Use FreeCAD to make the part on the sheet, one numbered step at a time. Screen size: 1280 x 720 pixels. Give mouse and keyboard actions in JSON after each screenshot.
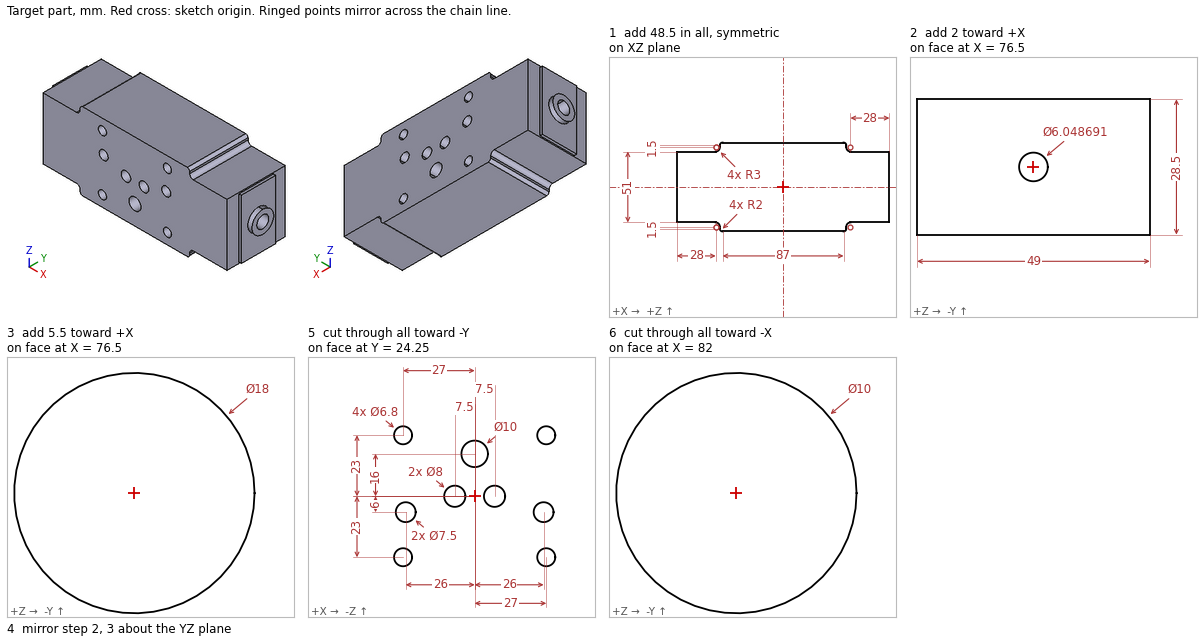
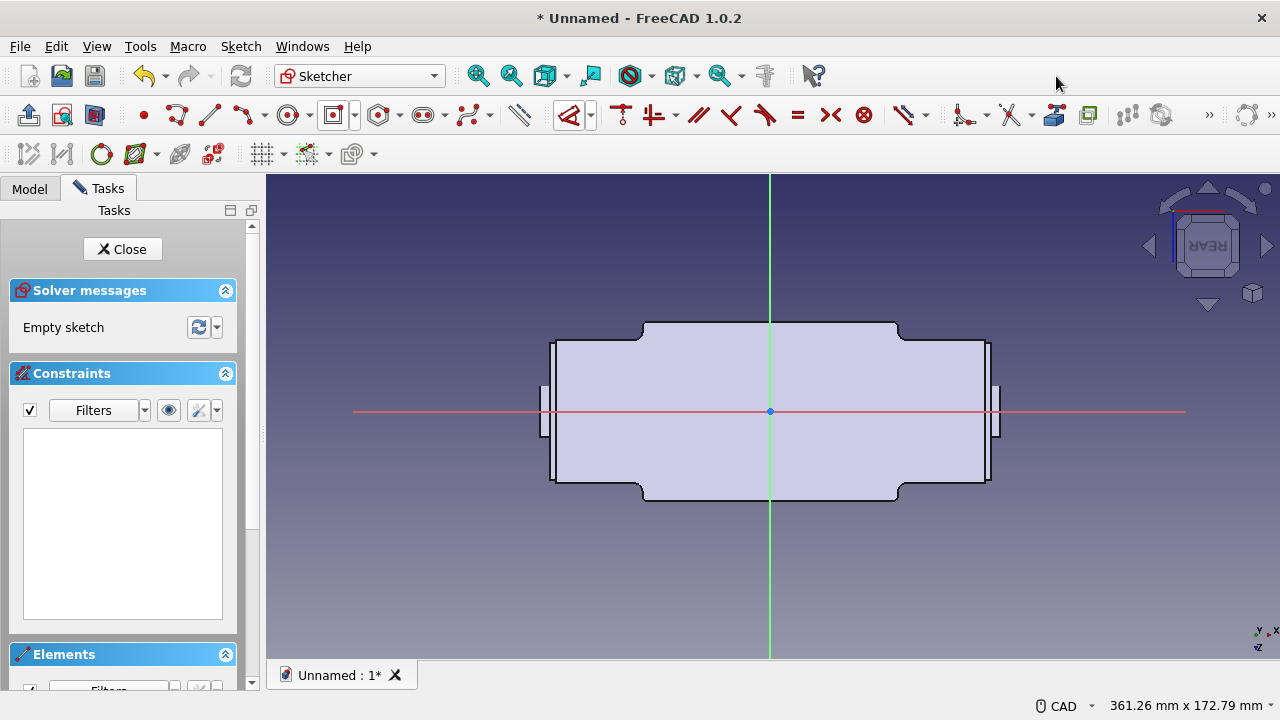
{"action": "scroll", "coordinate": [824, 408], "scroll_direction": "up", "scroll_amount": 4}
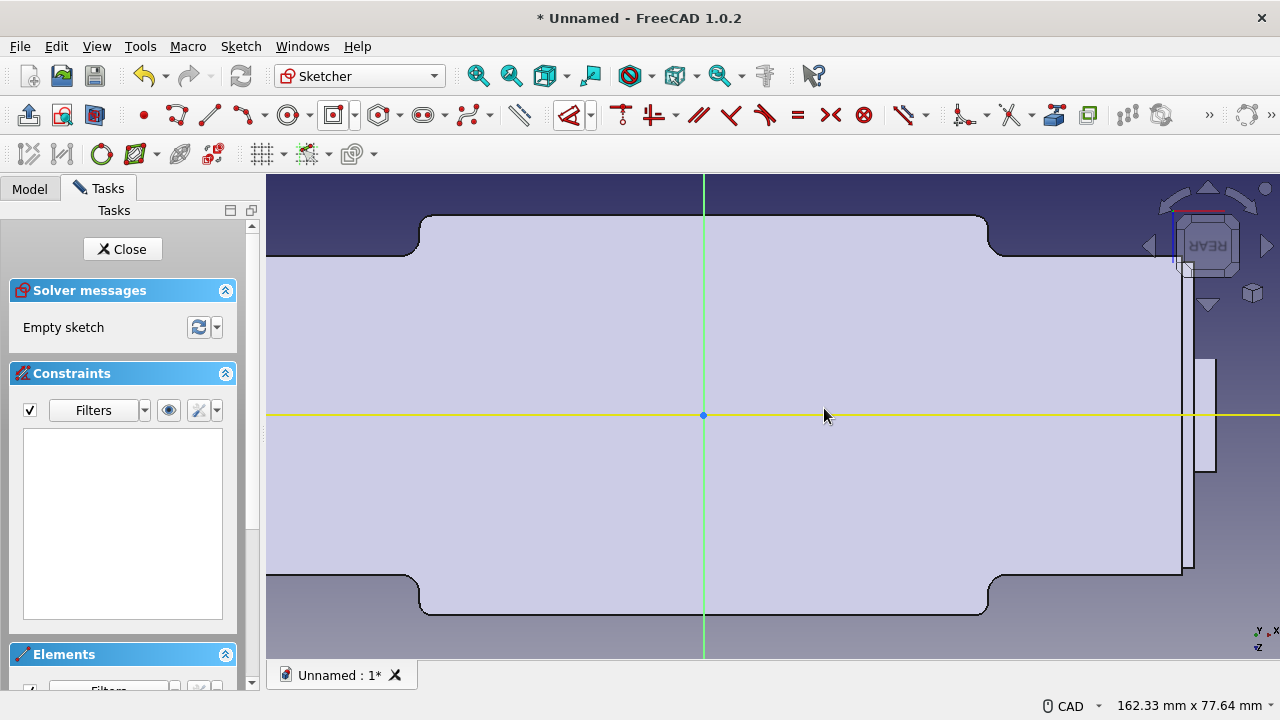
{"action": "key", "text": "g c"}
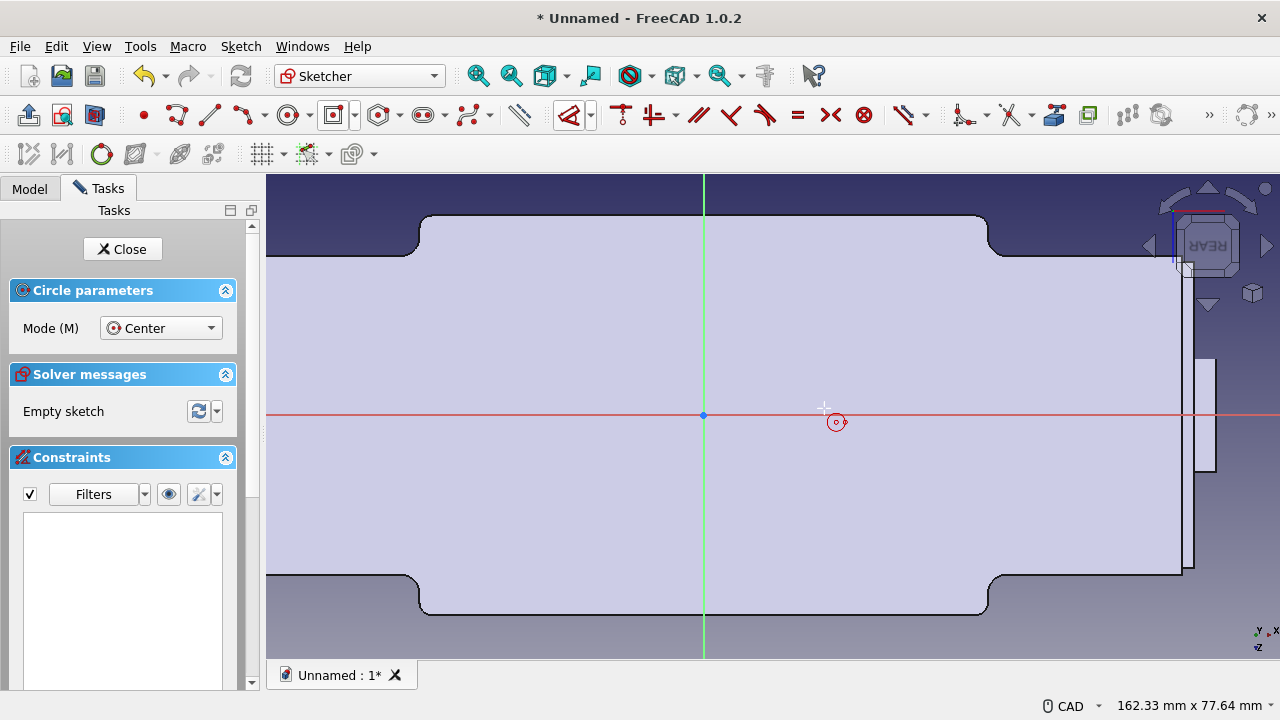
{"action": "left_click", "coordinate": [535, 272]}
{"action": "left_click", "coordinate": [550, 257]}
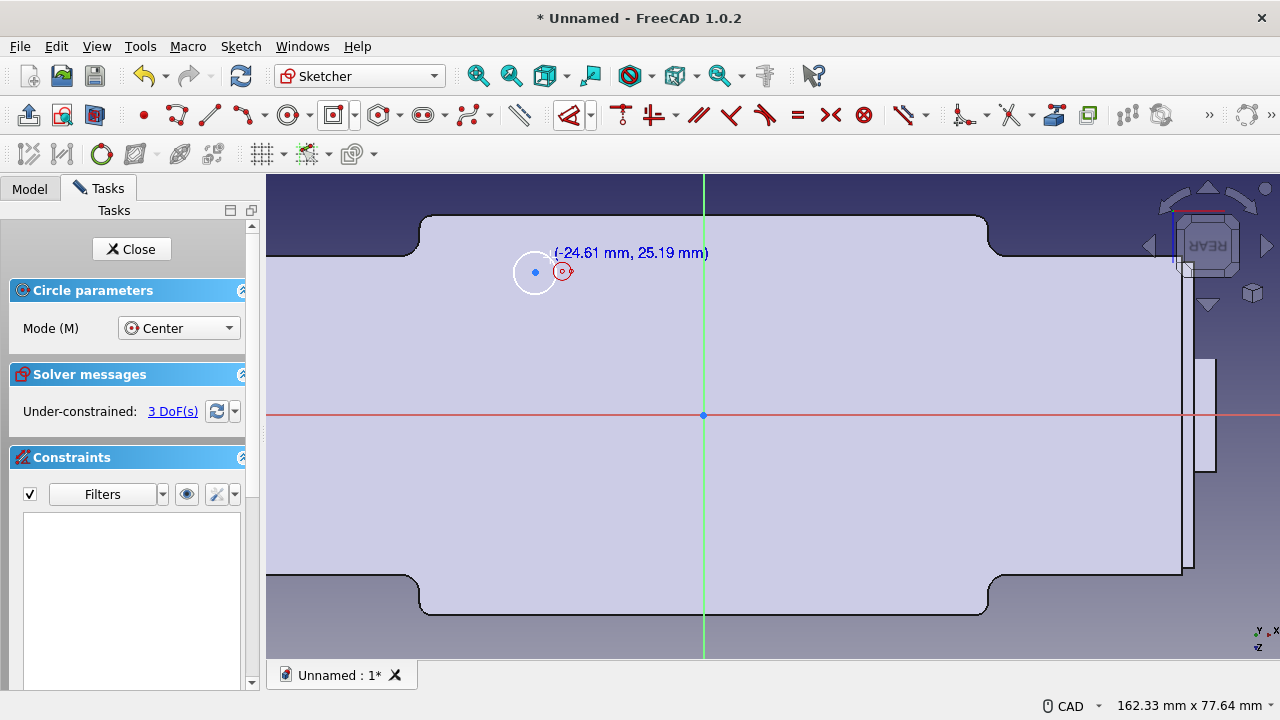
{"action": "left_click", "coordinate": [704, 315]}
{"action": "left_click", "coordinate": [726, 293]}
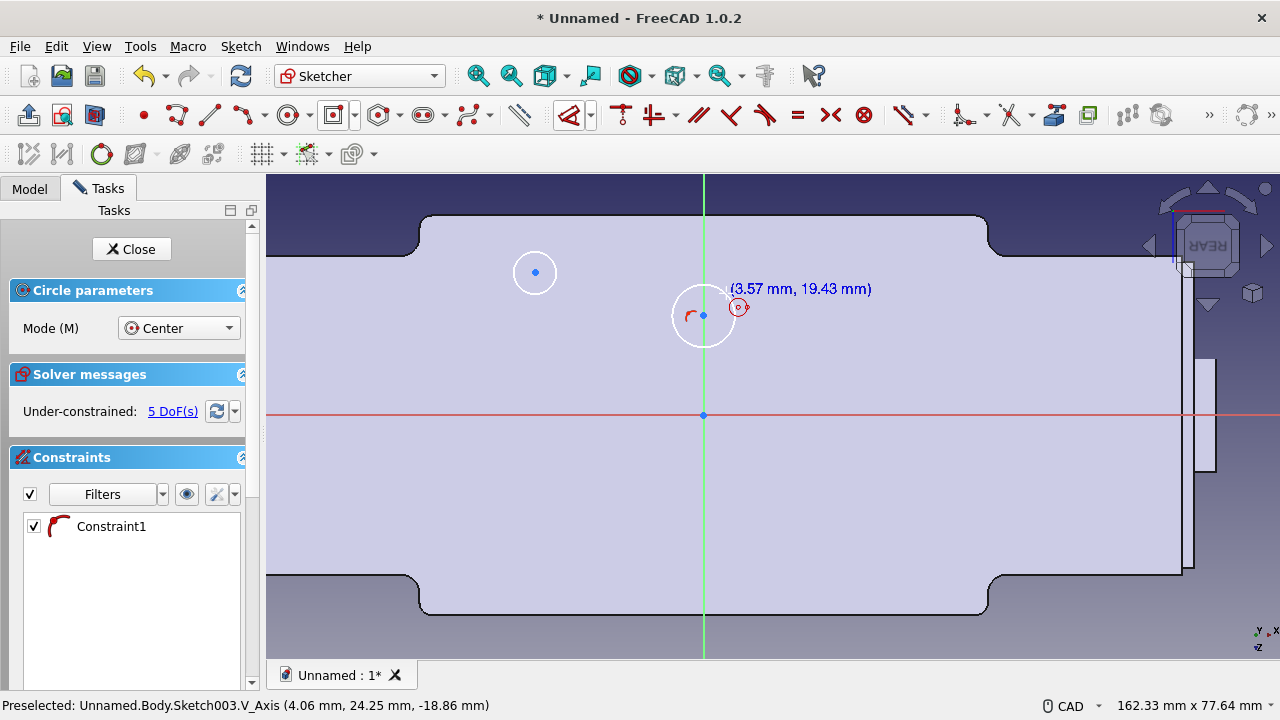
{"action": "left_click", "coordinate": [657, 415]}
{"action": "left_click", "coordinate": [675, 398]}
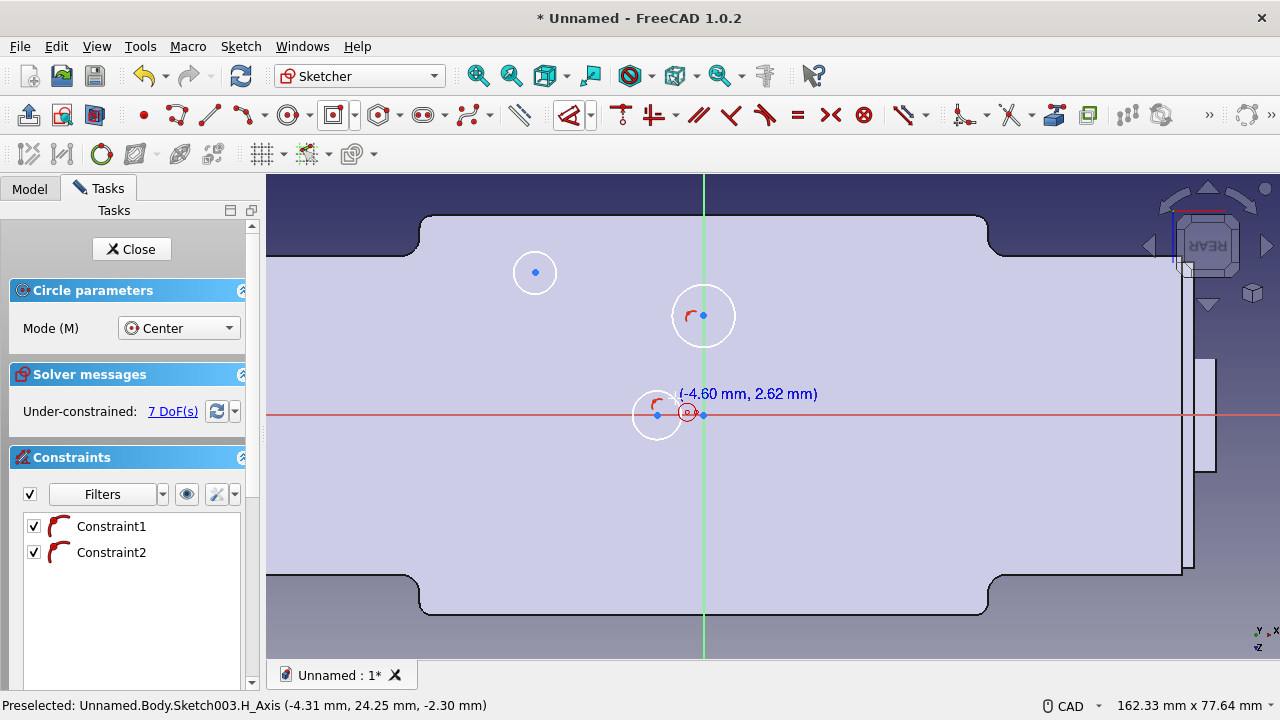
{"action": "left_click", "coordinate": [541, 453]}
{"action": "left_click", "coordinate": [558, 436]}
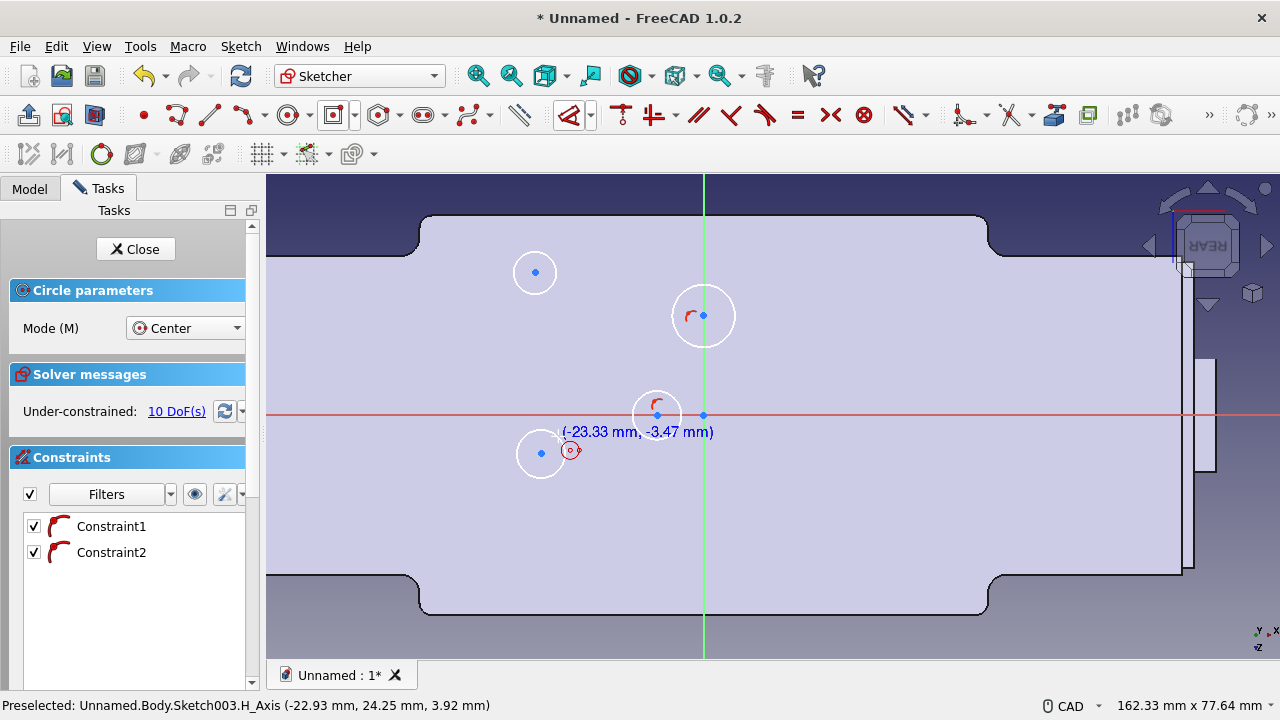
{"action": "left_click", "coordinate": [535, 559]}
{"action": "left_click", "coordinate": [550, 544]}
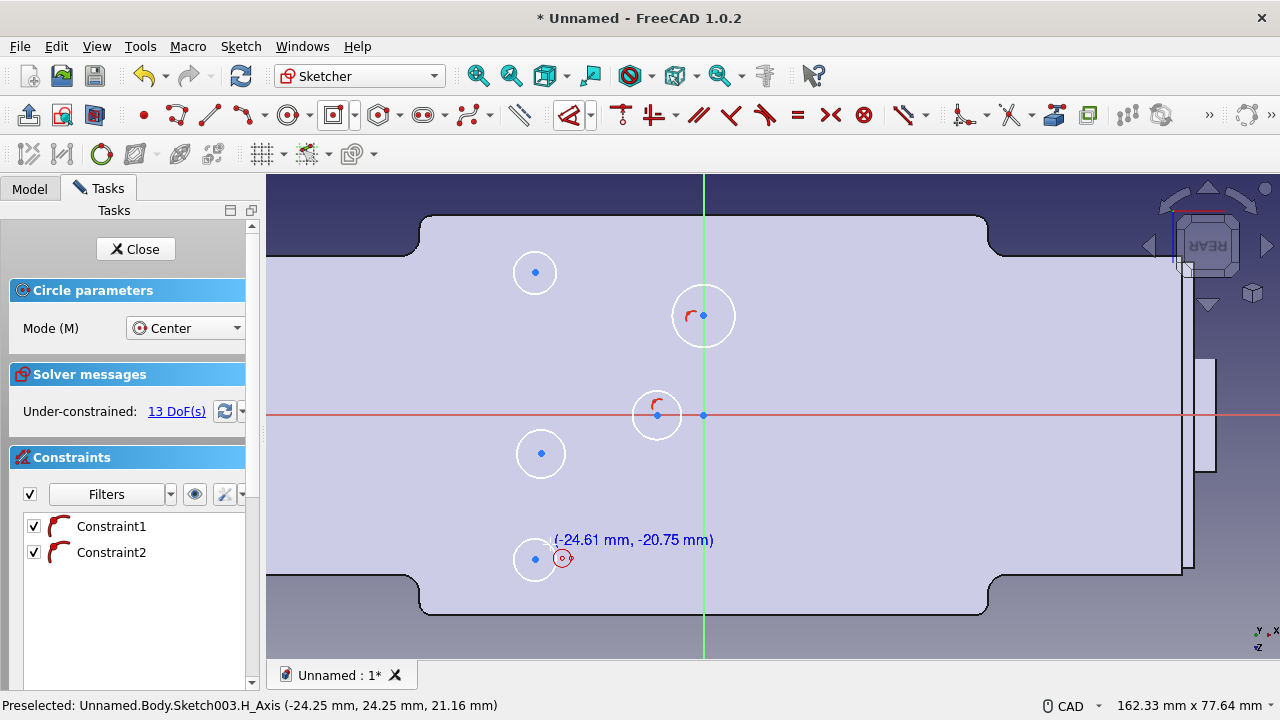
{"action": "left_click", "coordinate": [751, 415]}
{"action": "left_click", "coordinate": [768, 398]}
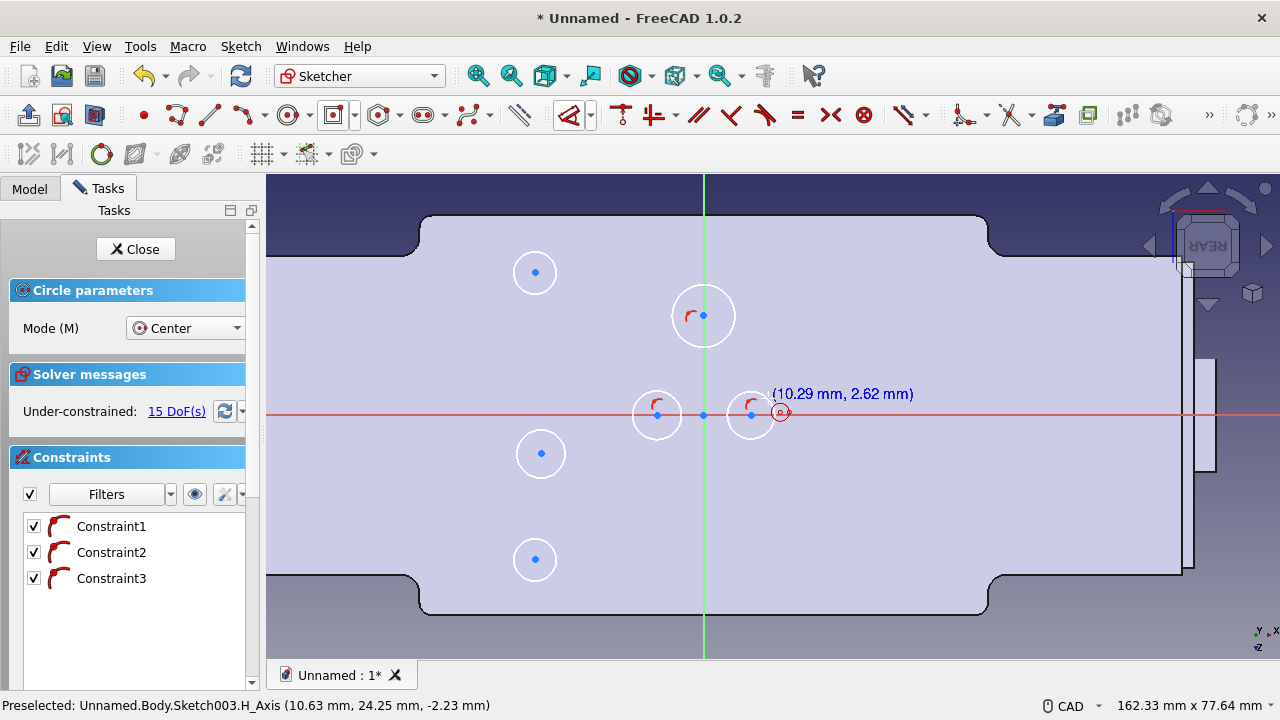
{"action": "left_click", "coordinate": [872, 559]}
{"action": "left_click", "coordinate": [887, 544]}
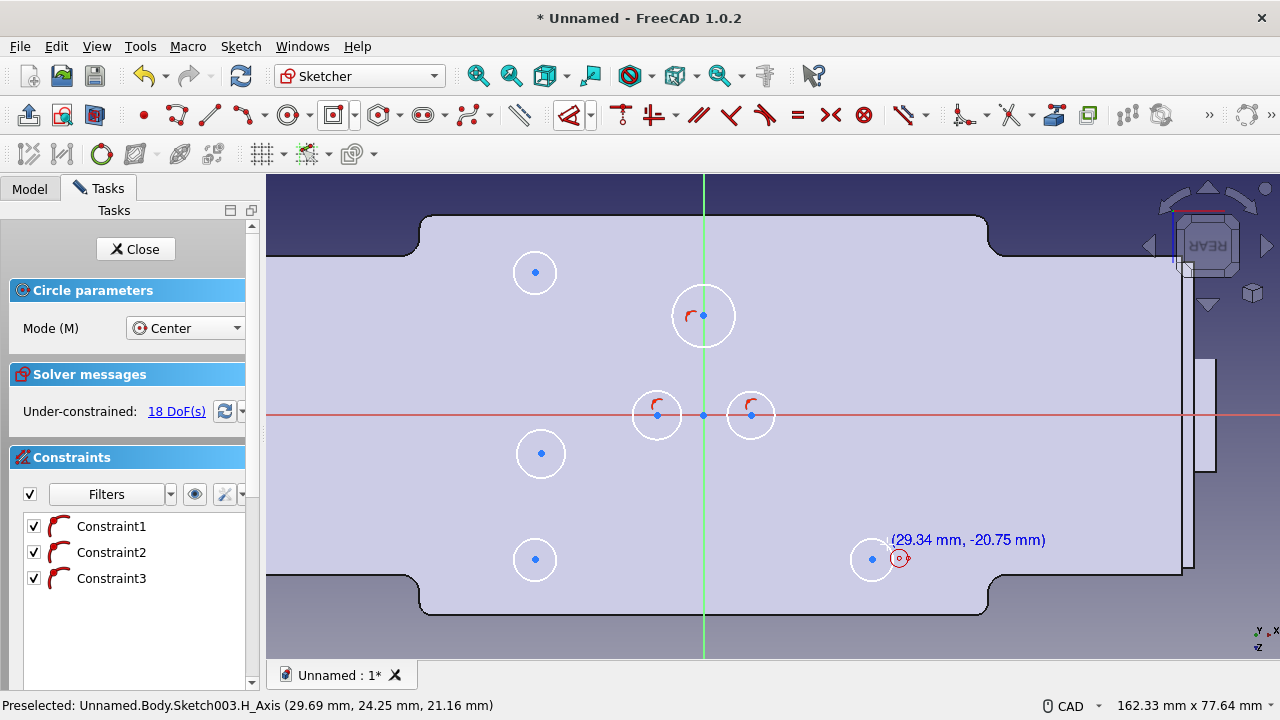
{"action": "left_click", "coordinate": [866, 453]}
{"action": "left_click", "coordinate": [883, 436]}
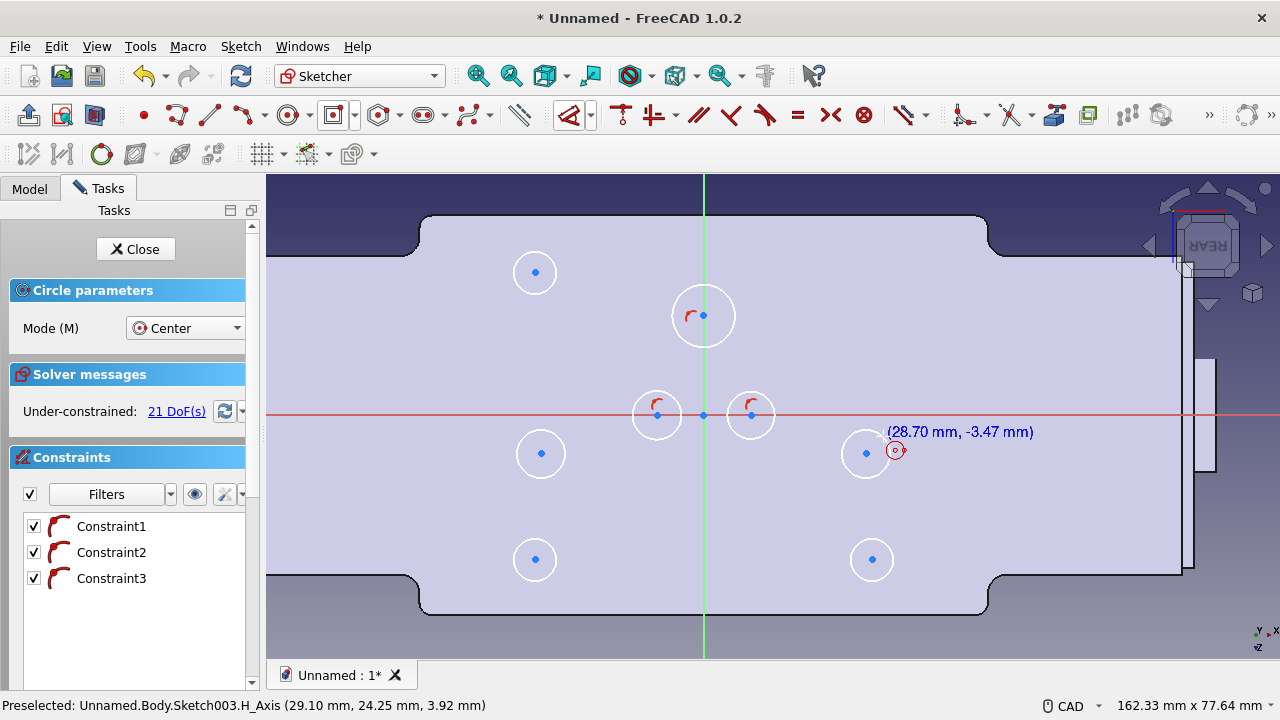
{"action": "left_click", "coordinate": [872, 272]}
{"action": "left_click", "coordinate": [887, 257]}
{"action": "key", "text": "Escape"}